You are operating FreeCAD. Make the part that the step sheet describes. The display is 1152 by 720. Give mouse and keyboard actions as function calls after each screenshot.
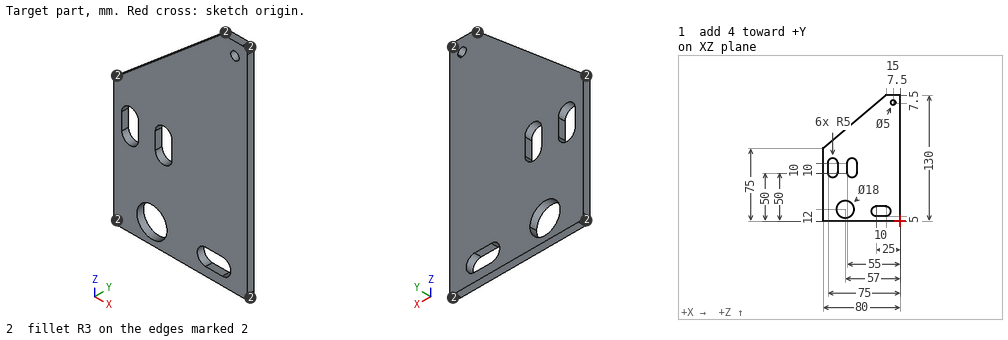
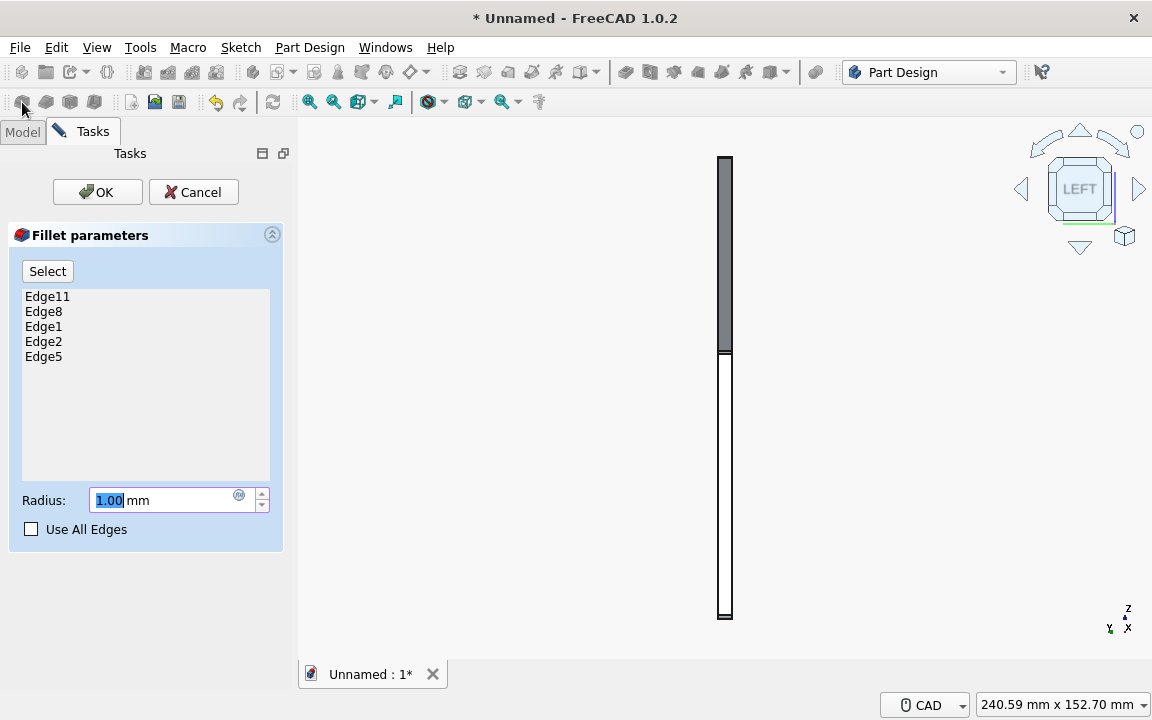
text(3)
key(Tab)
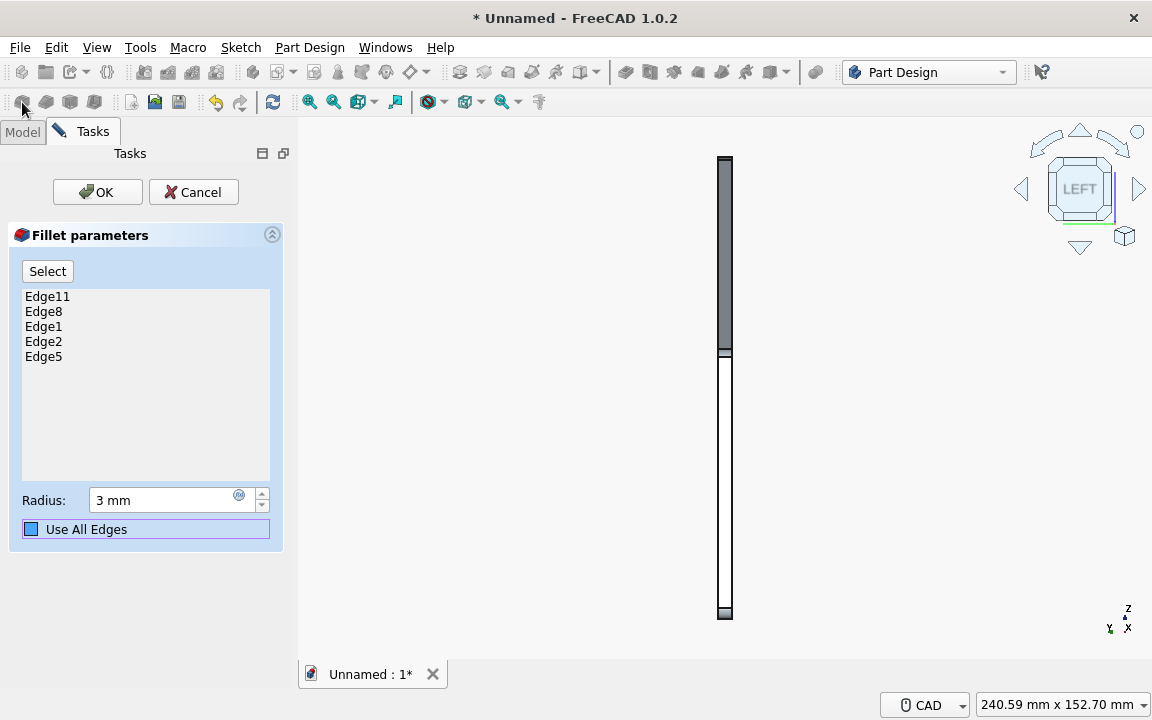
click(98, 192)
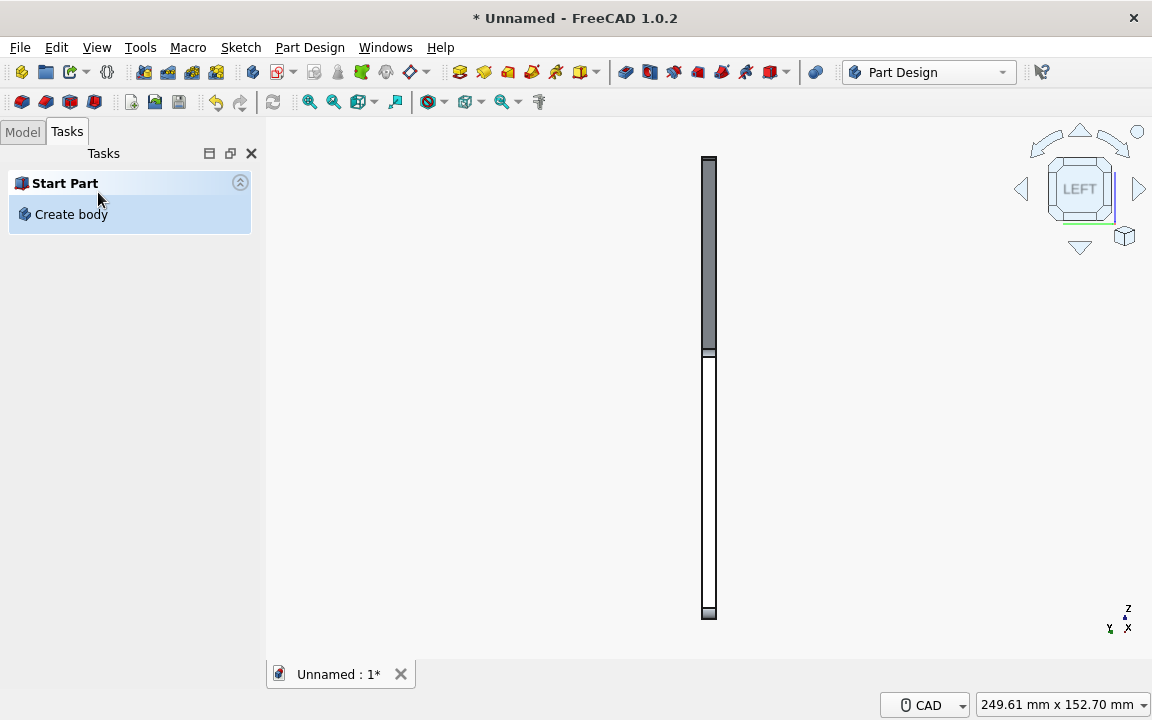
key(0)